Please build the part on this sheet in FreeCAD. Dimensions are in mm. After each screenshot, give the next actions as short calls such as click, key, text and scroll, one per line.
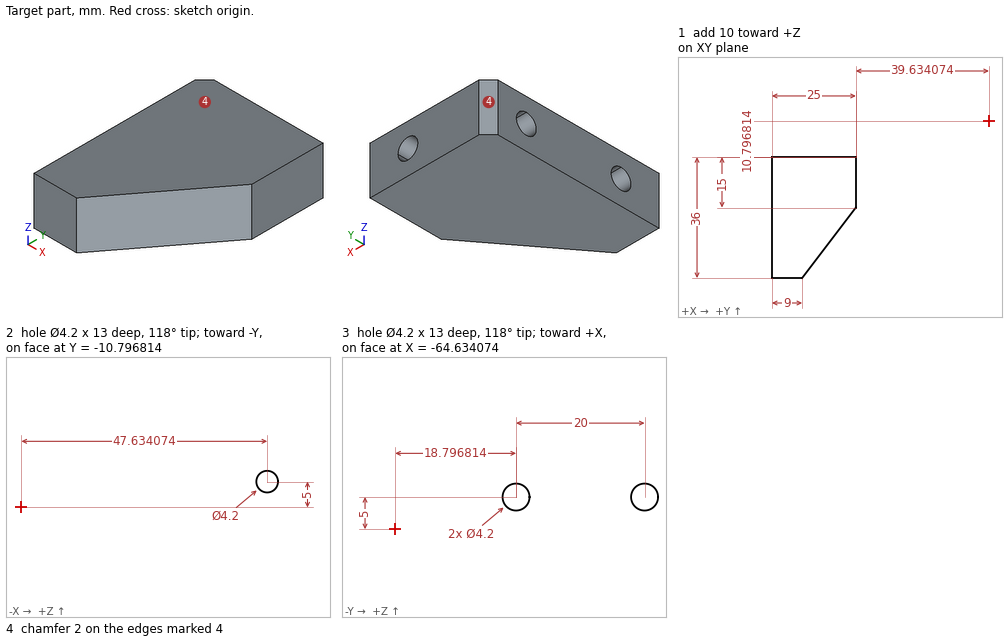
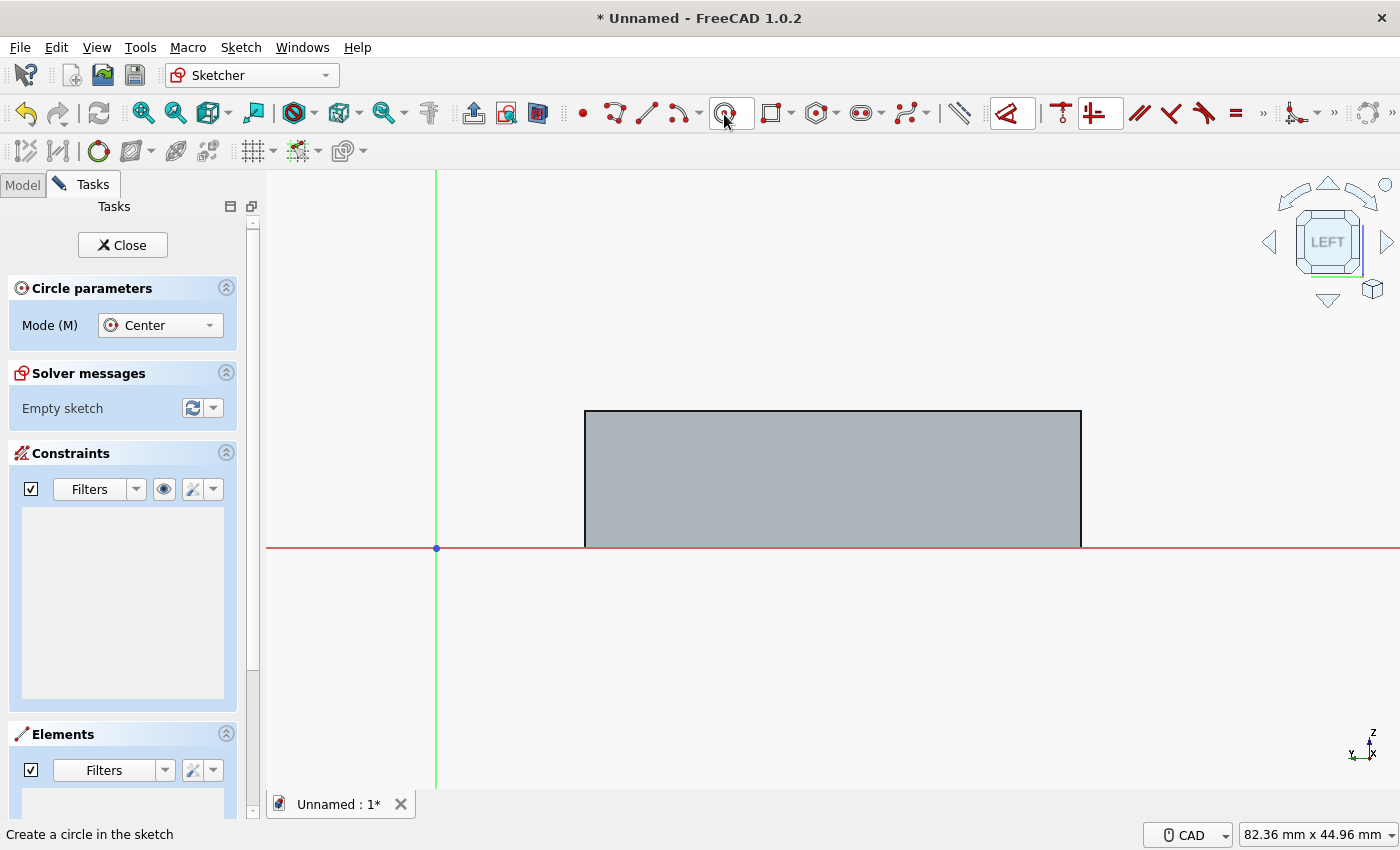
click(695, 480)
move(716, 459)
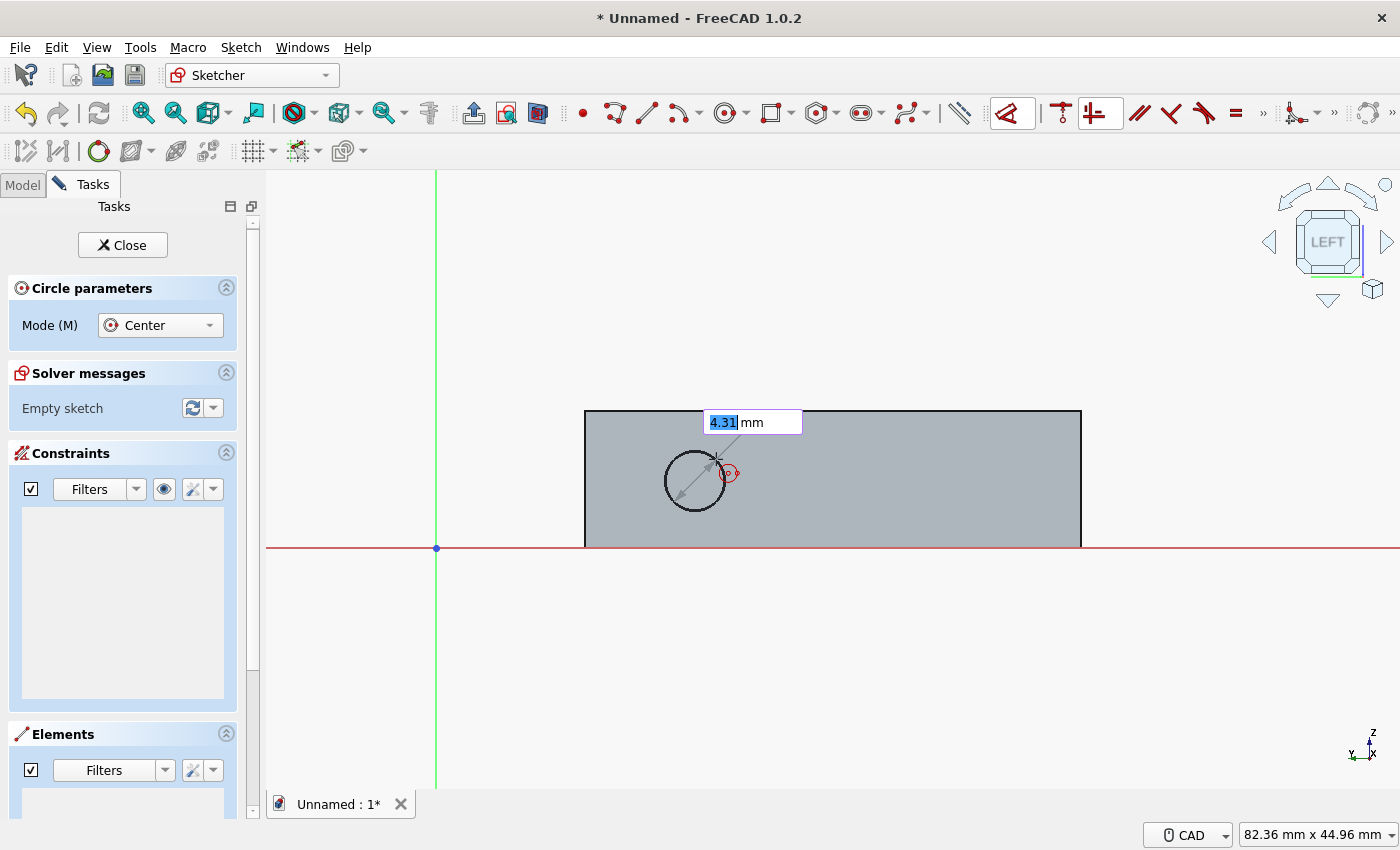
text(4.2)
key(Return)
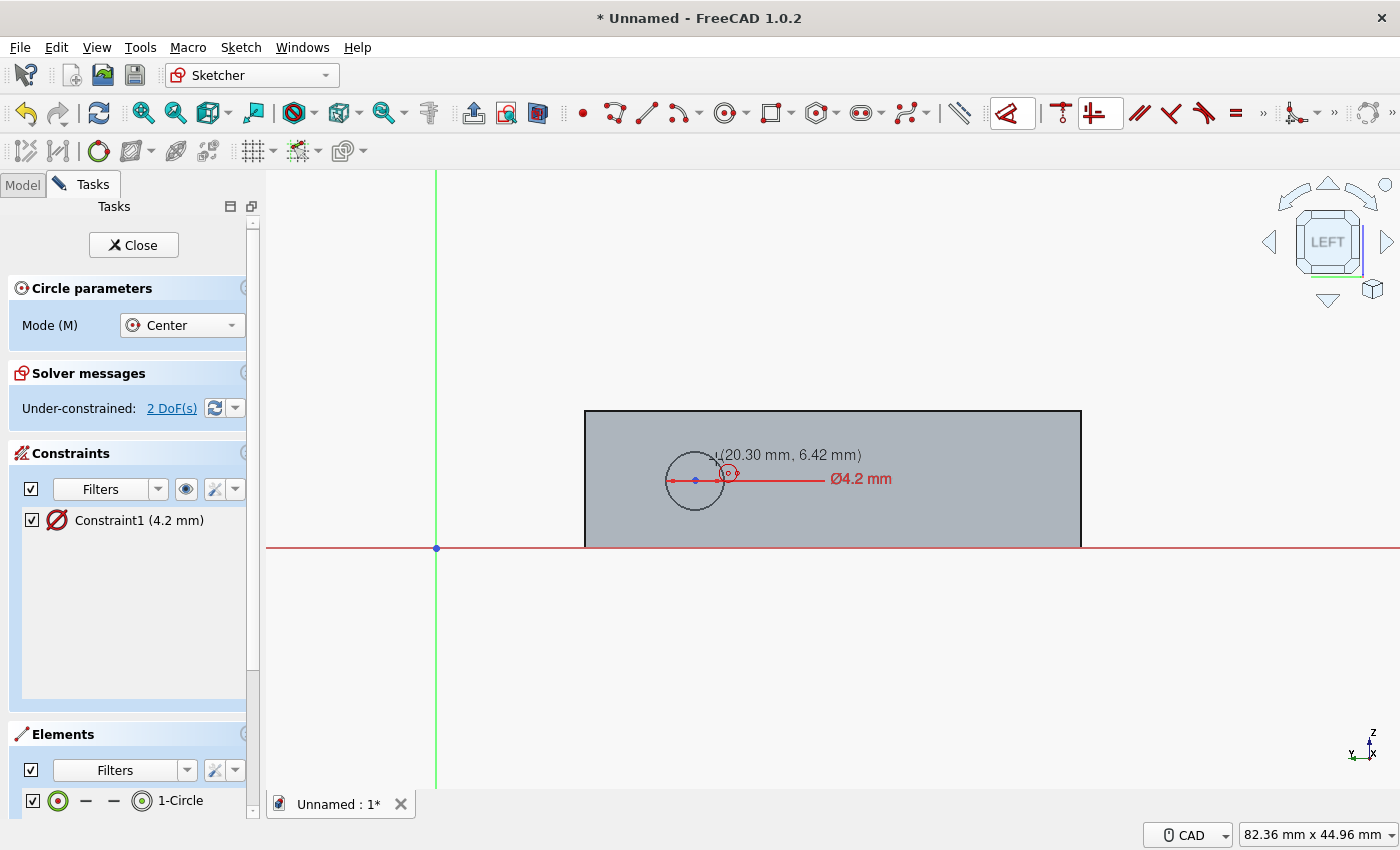
click(971, 480)
move(991, 459)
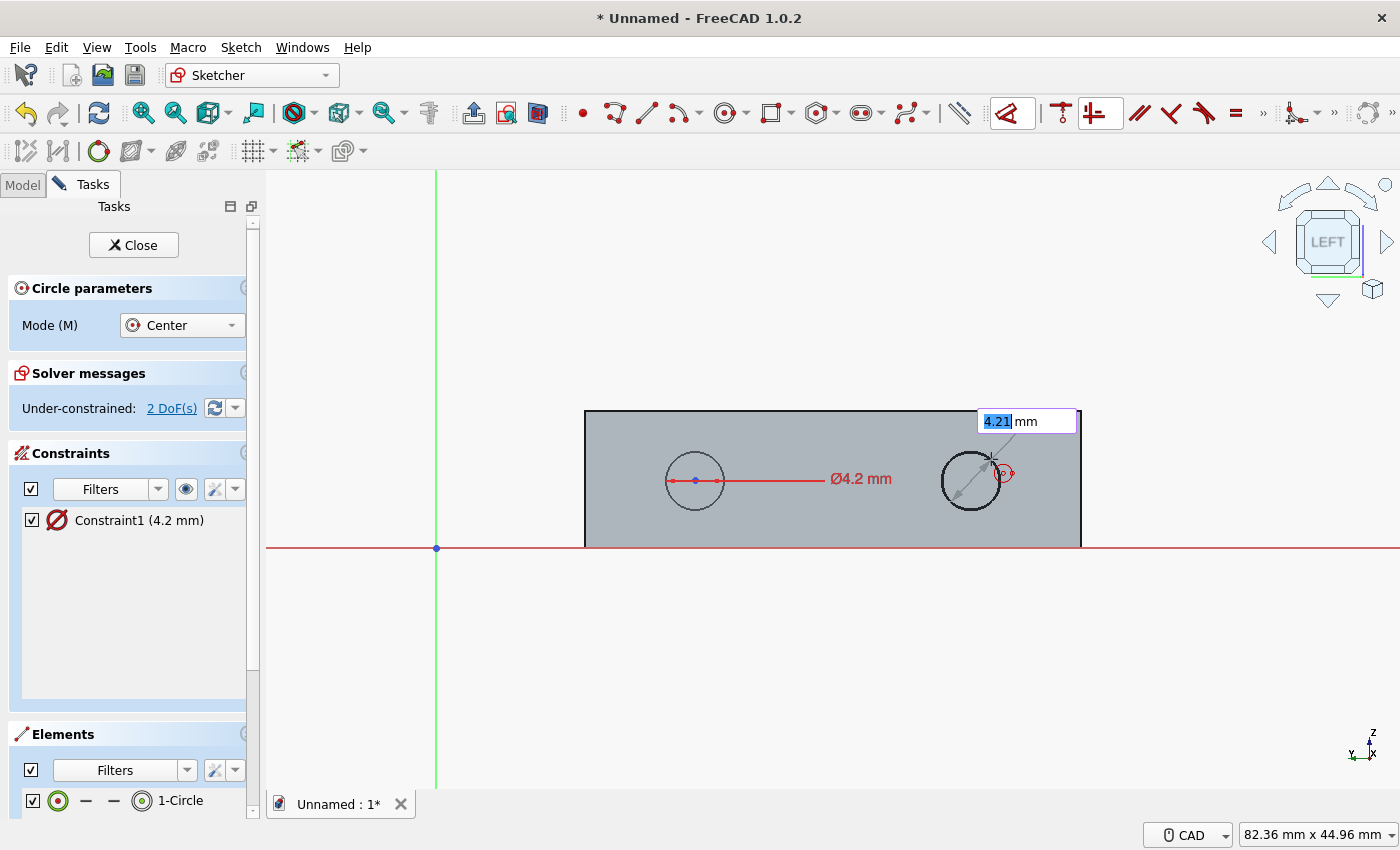
text(4.2)
key(Return)
key(Escape)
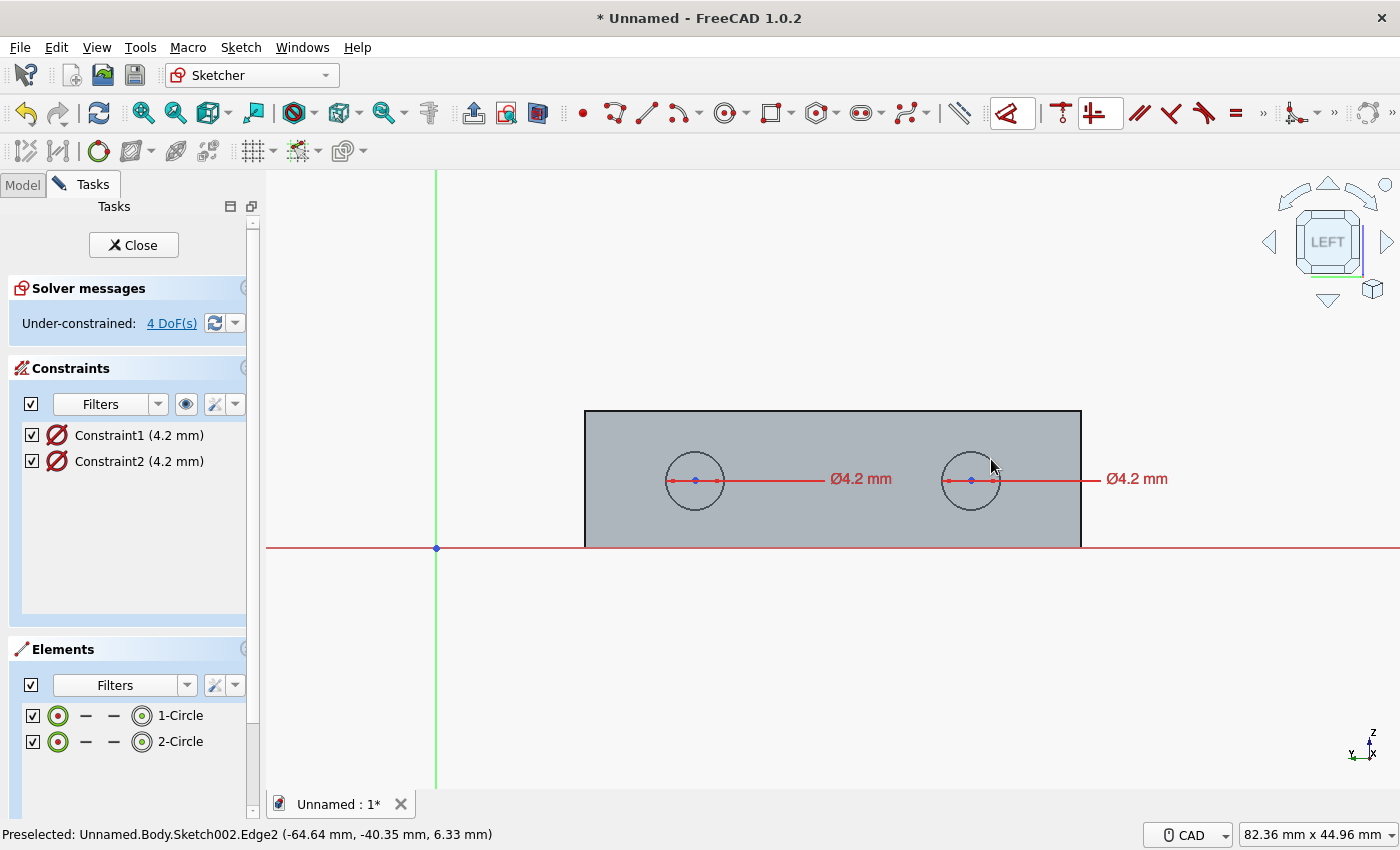
click(695, 481)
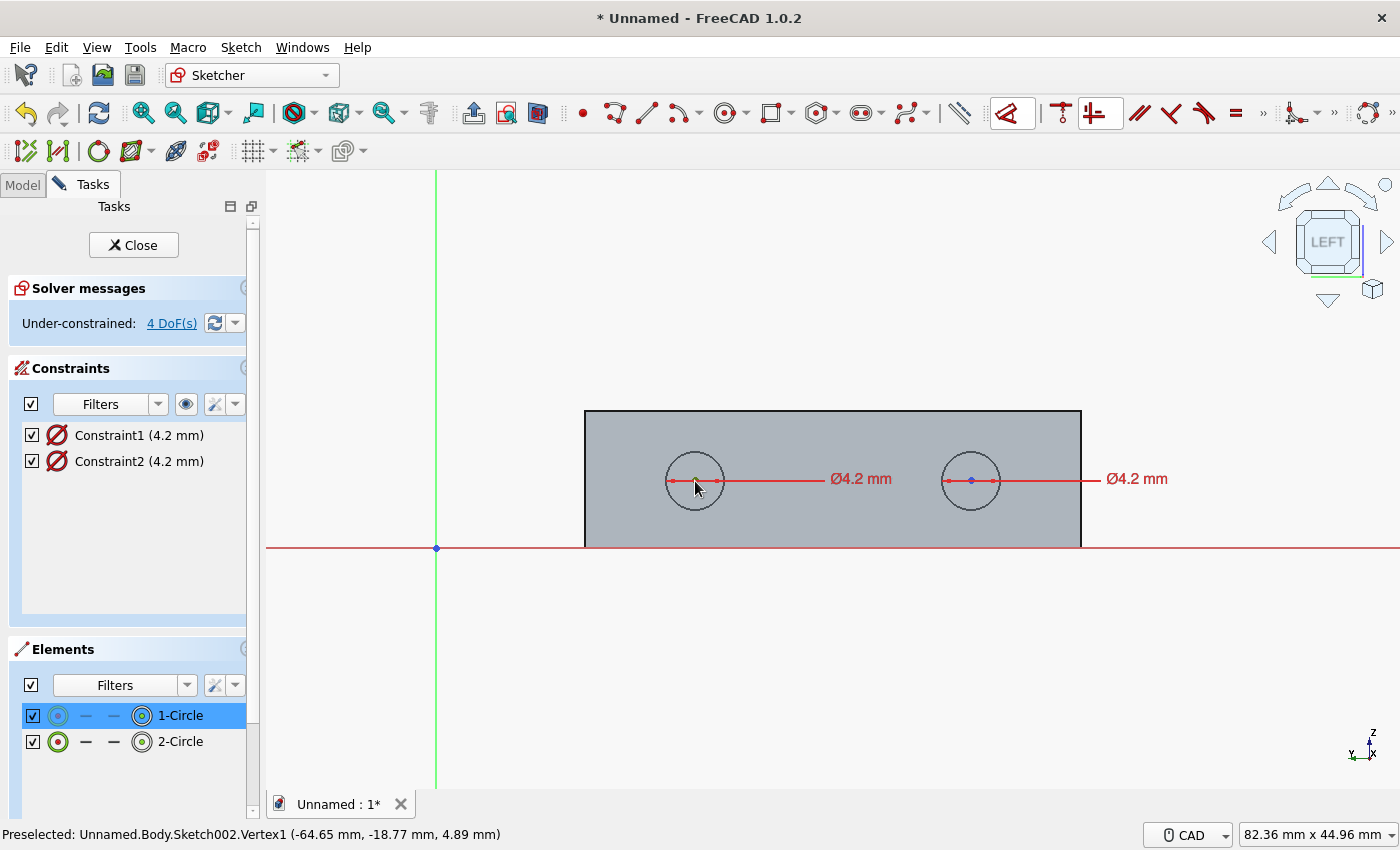
click(971, 481)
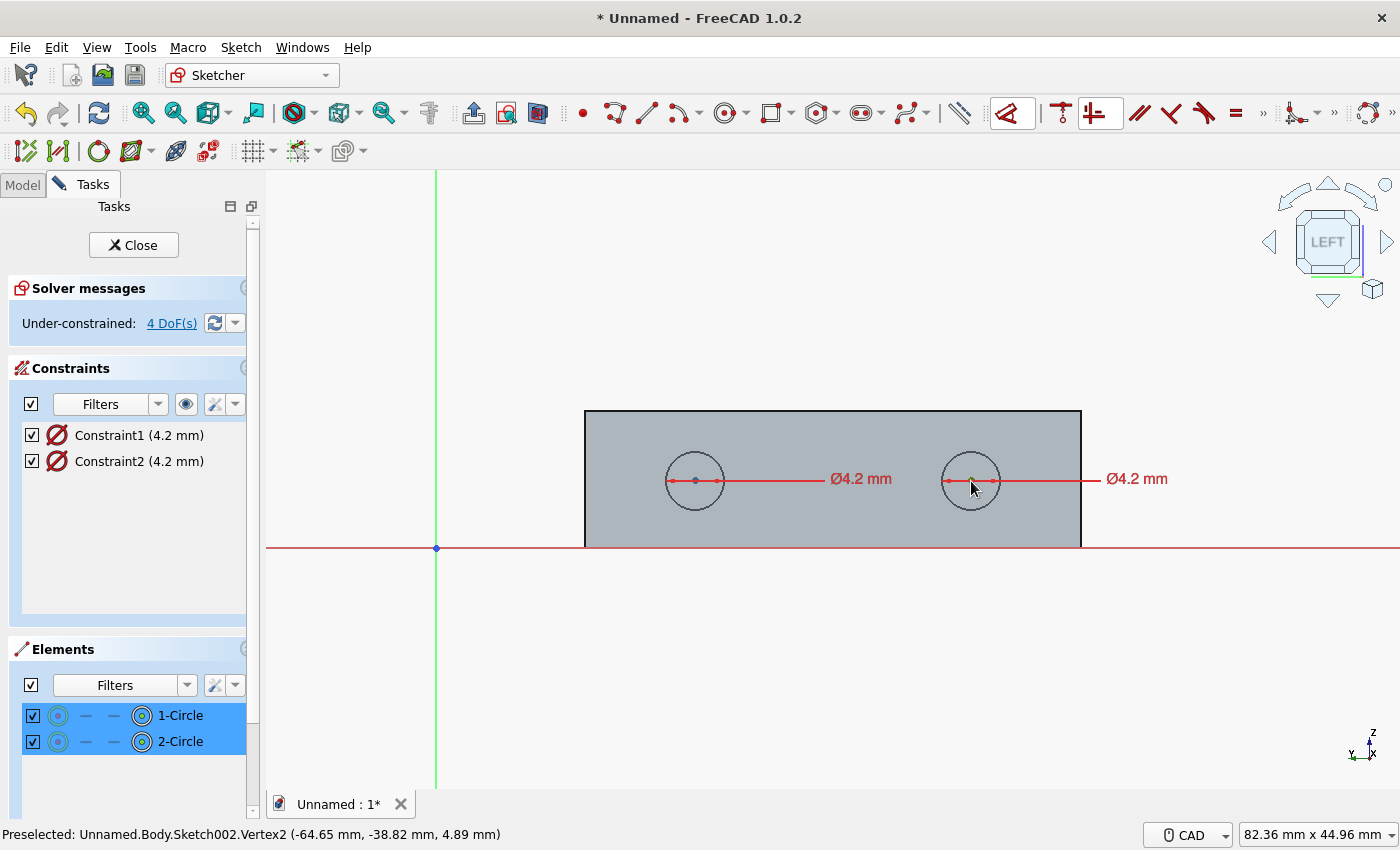
key(h)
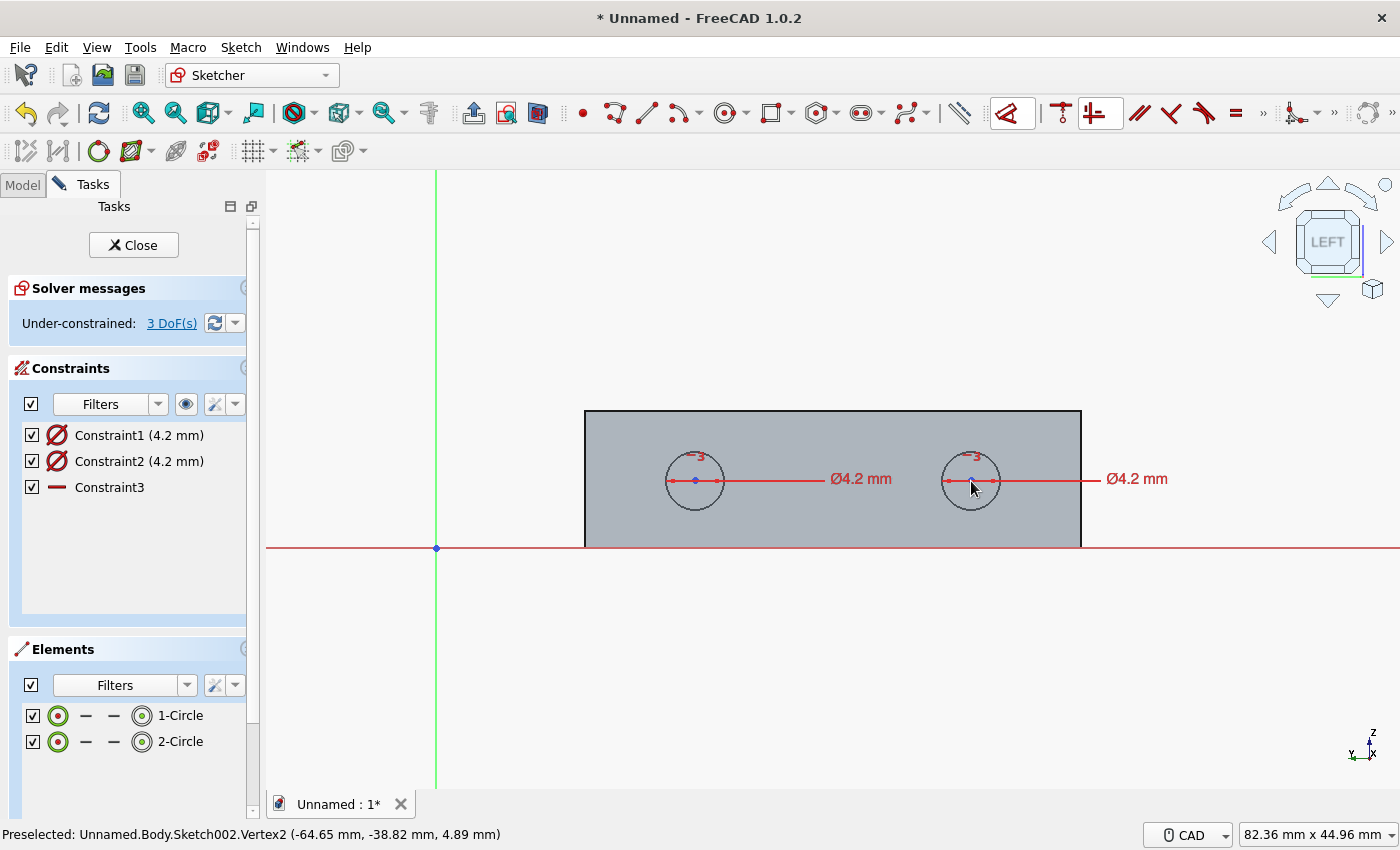
click(695, 481)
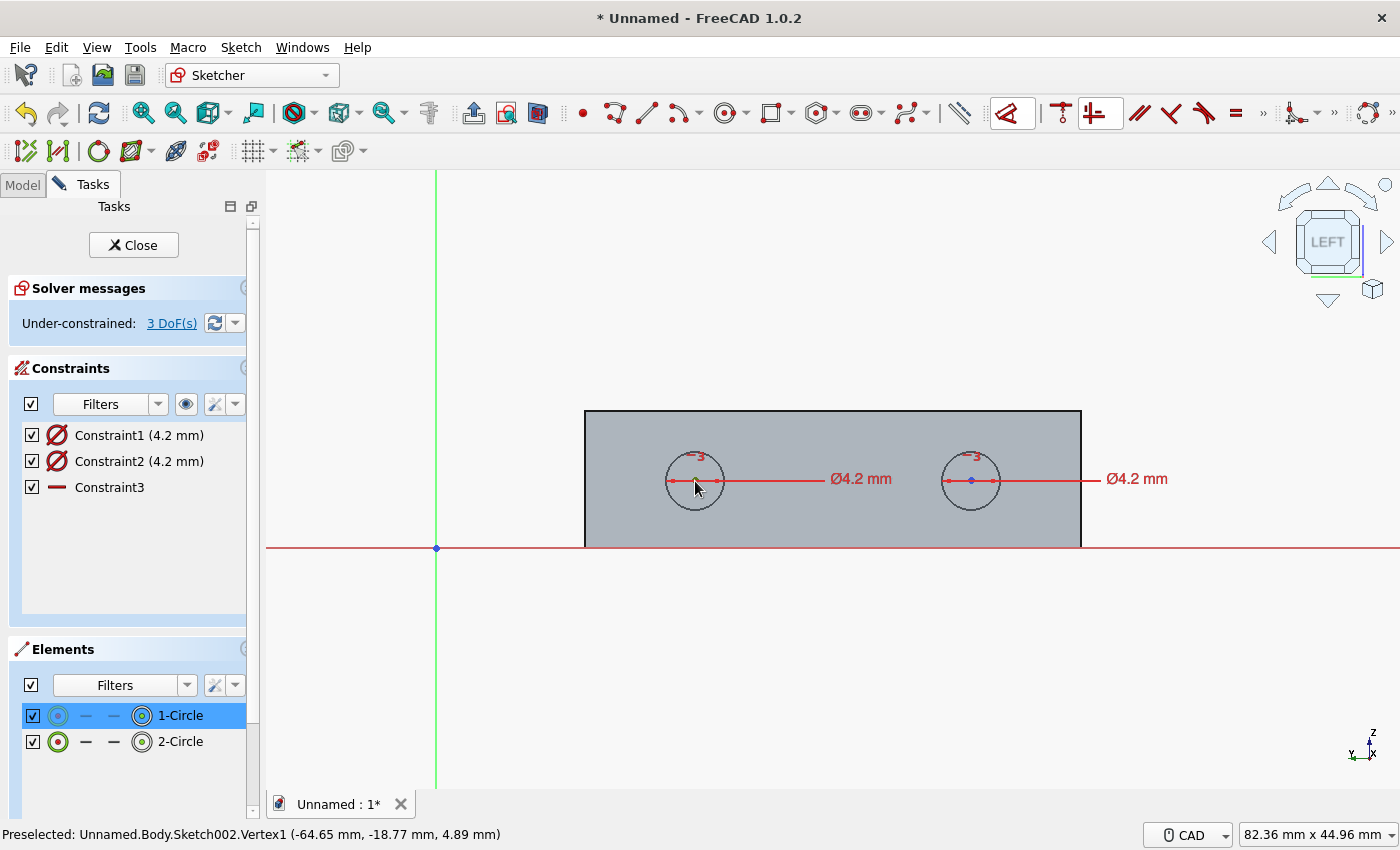
click(1030, 114)